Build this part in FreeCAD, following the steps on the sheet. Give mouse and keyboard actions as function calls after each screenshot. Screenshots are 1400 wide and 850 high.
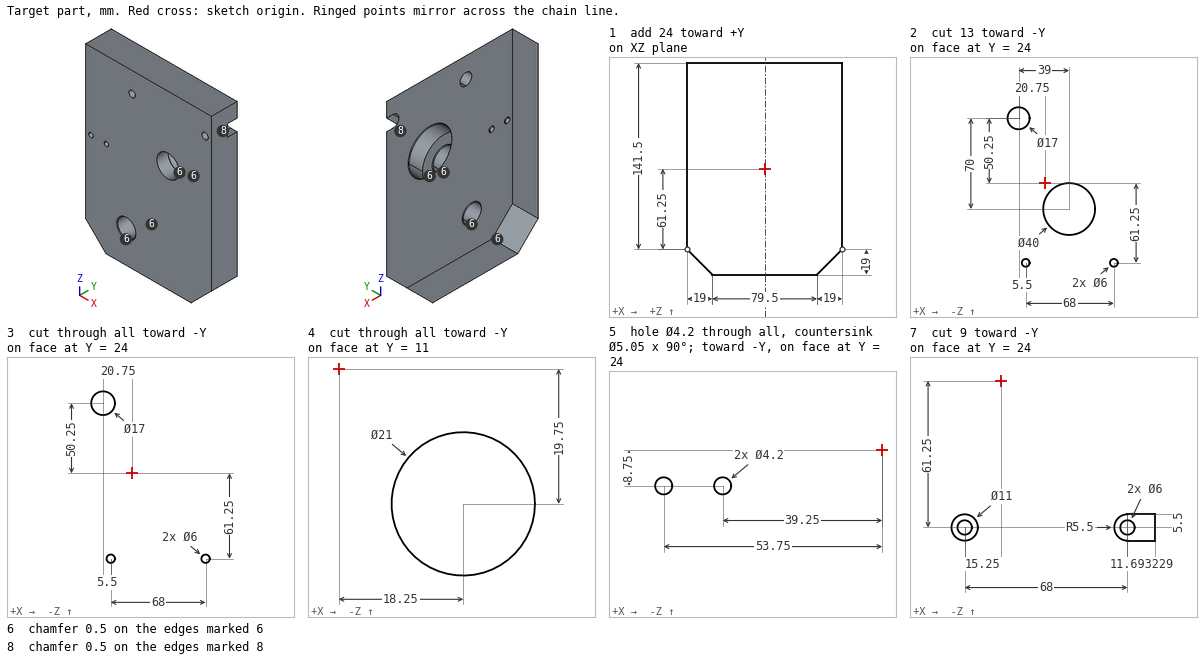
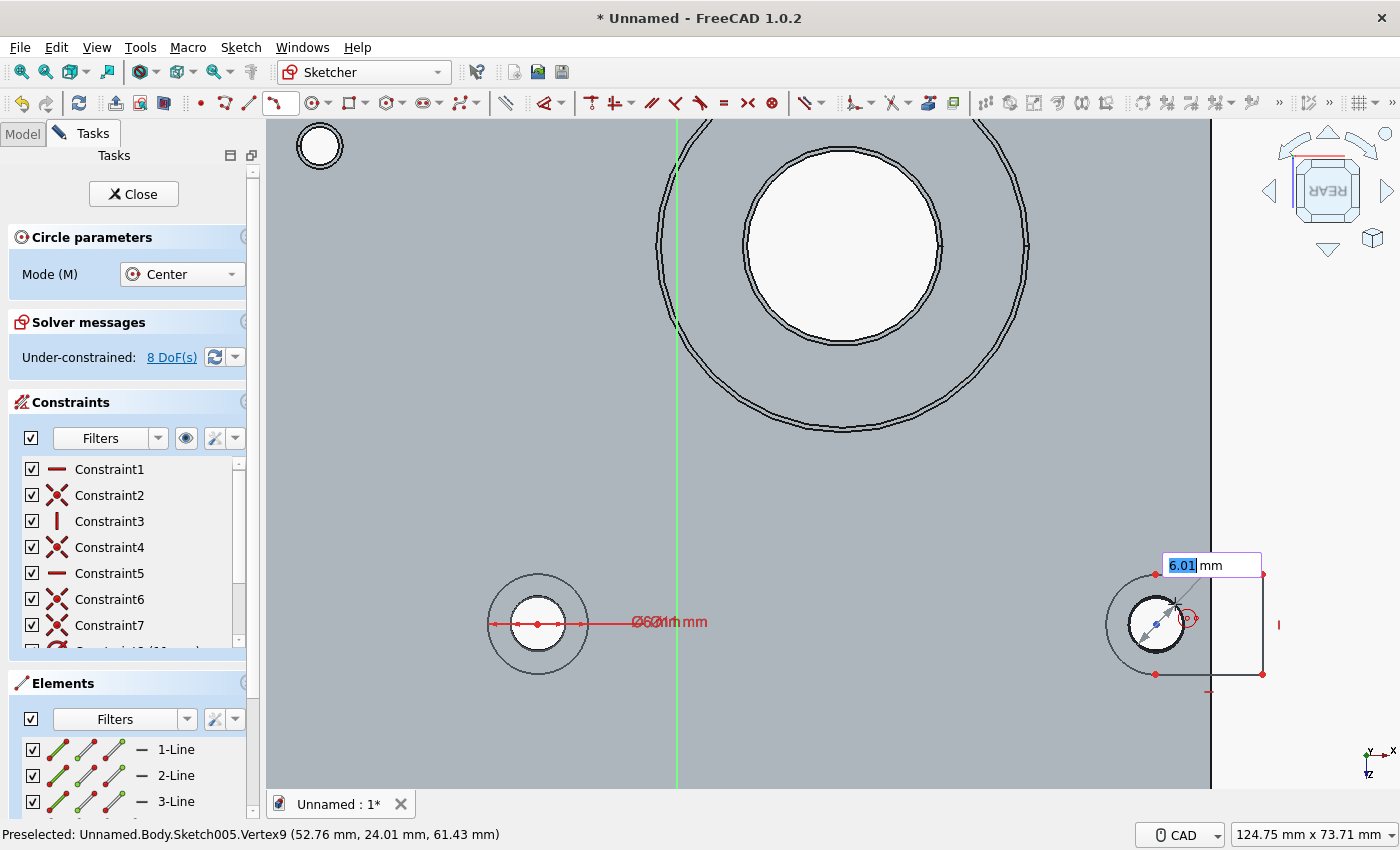
text(6)
key(Return)
key(Escape)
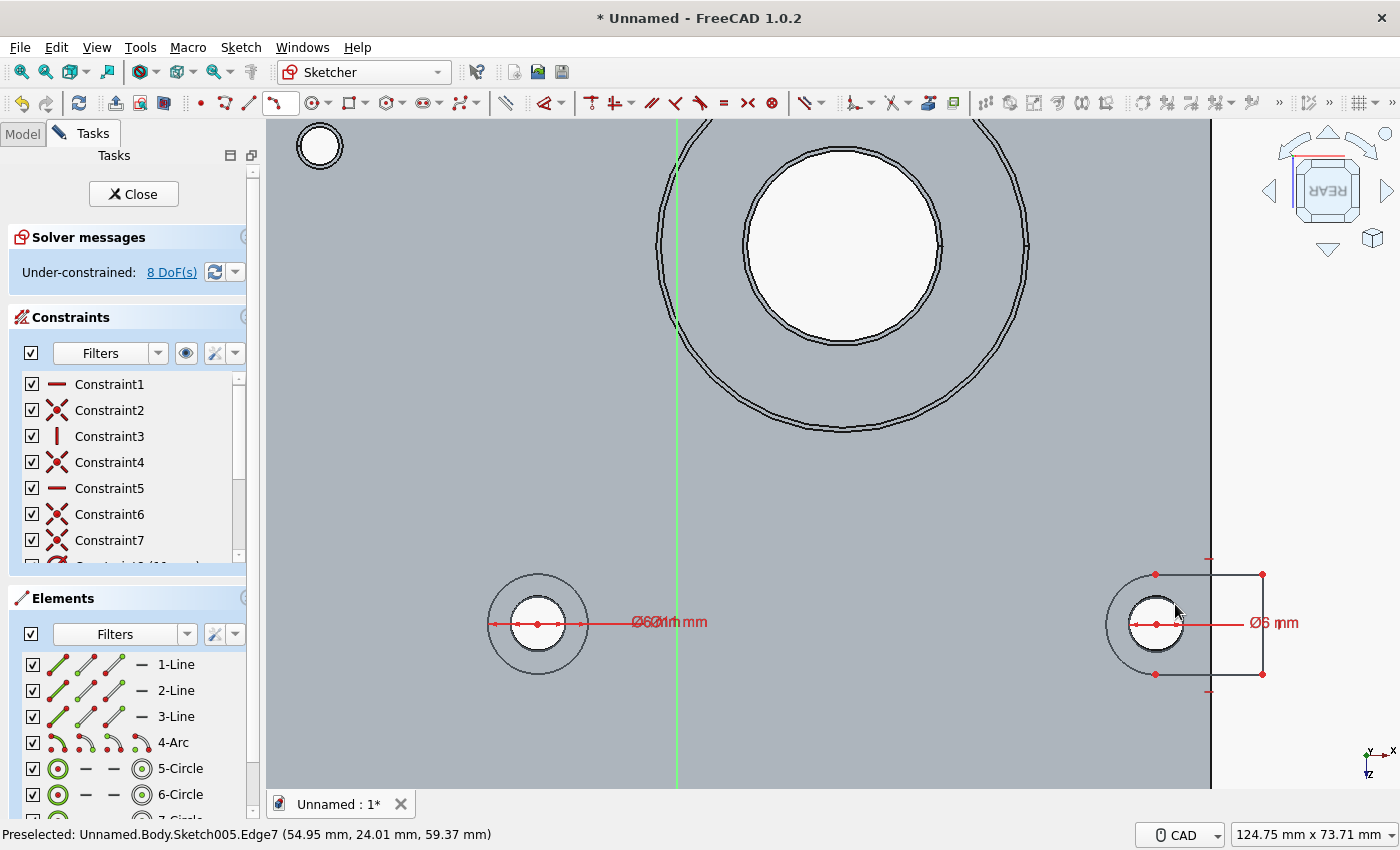
click(1188, 575)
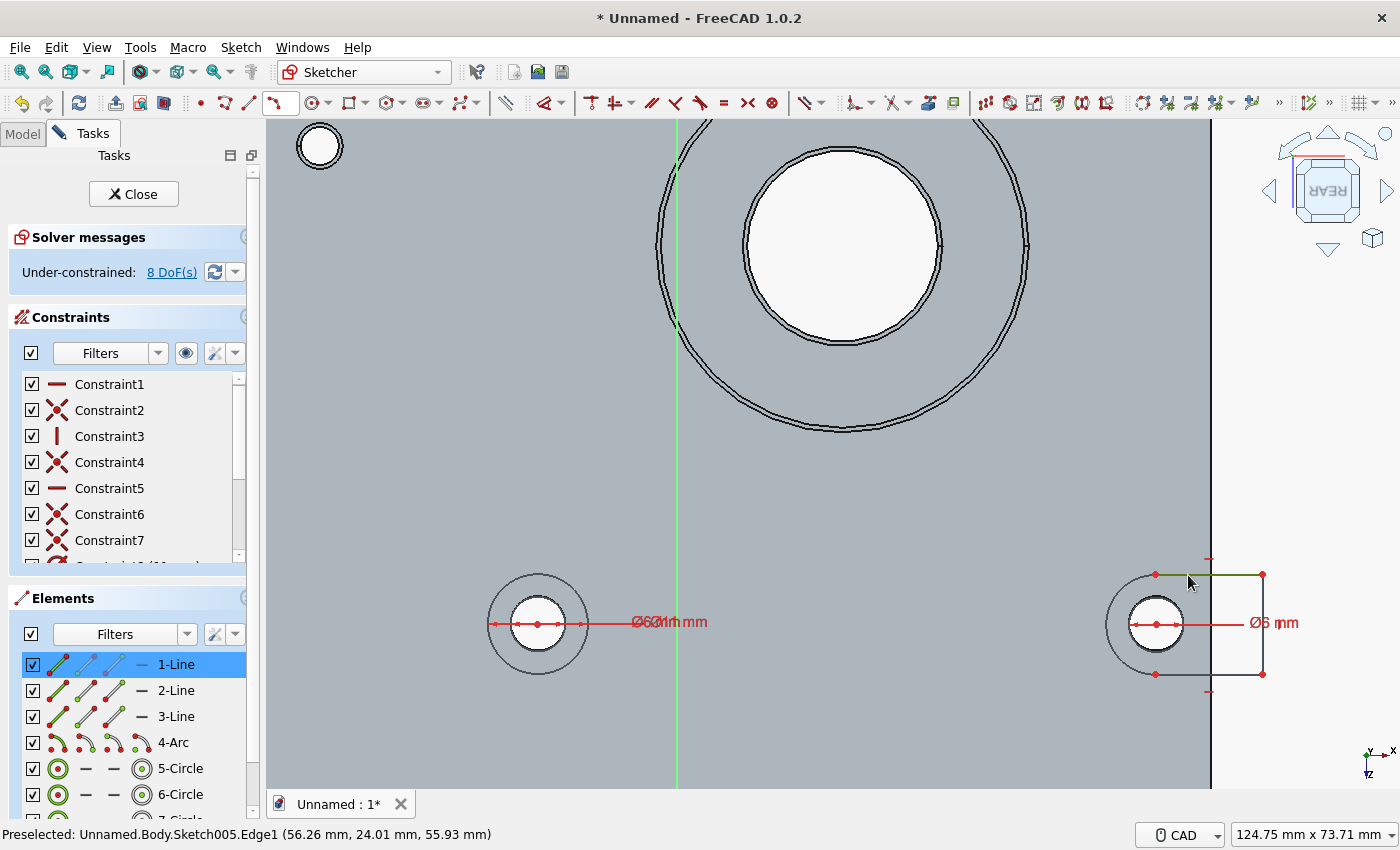
click(1116, 596)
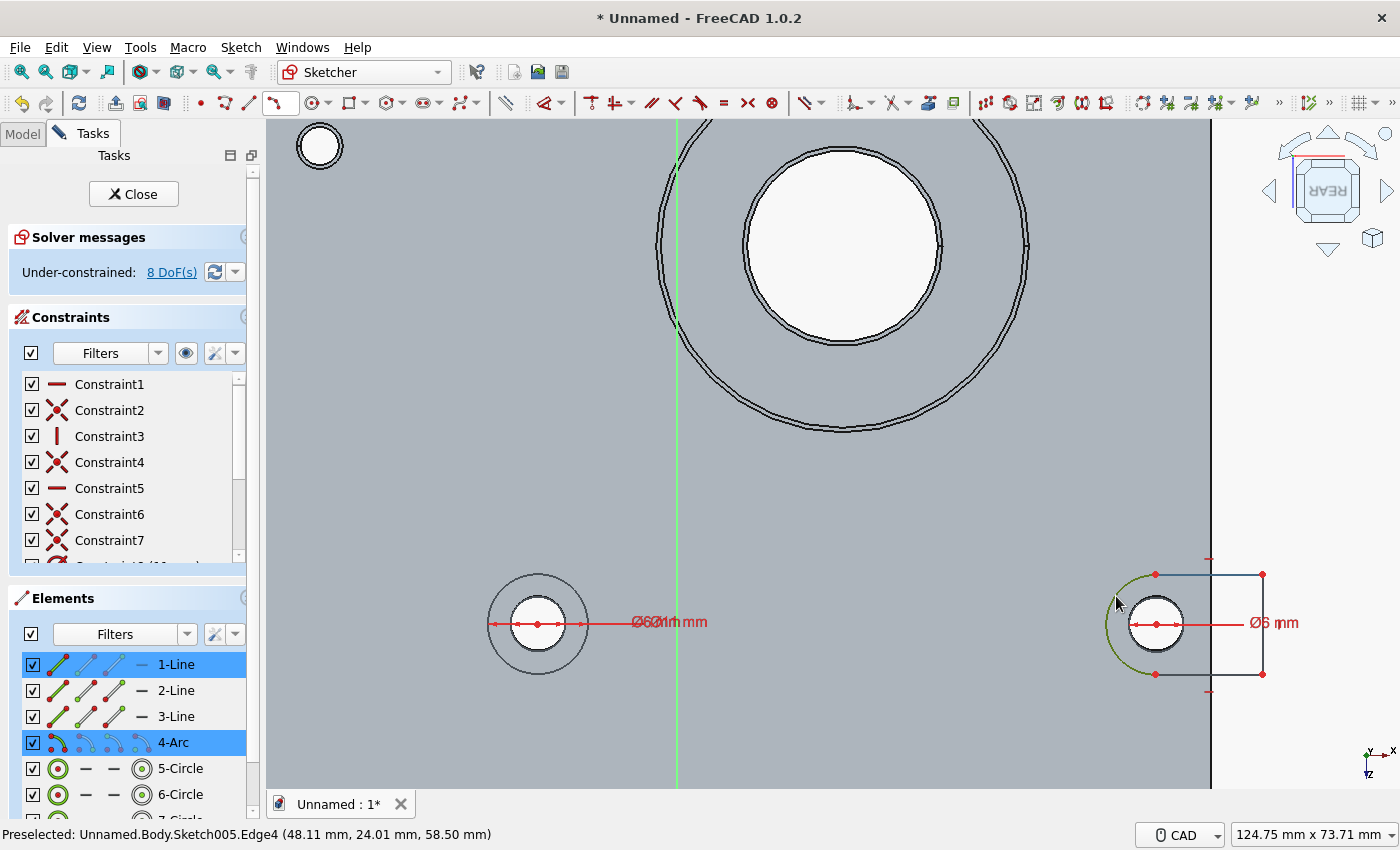
key(t)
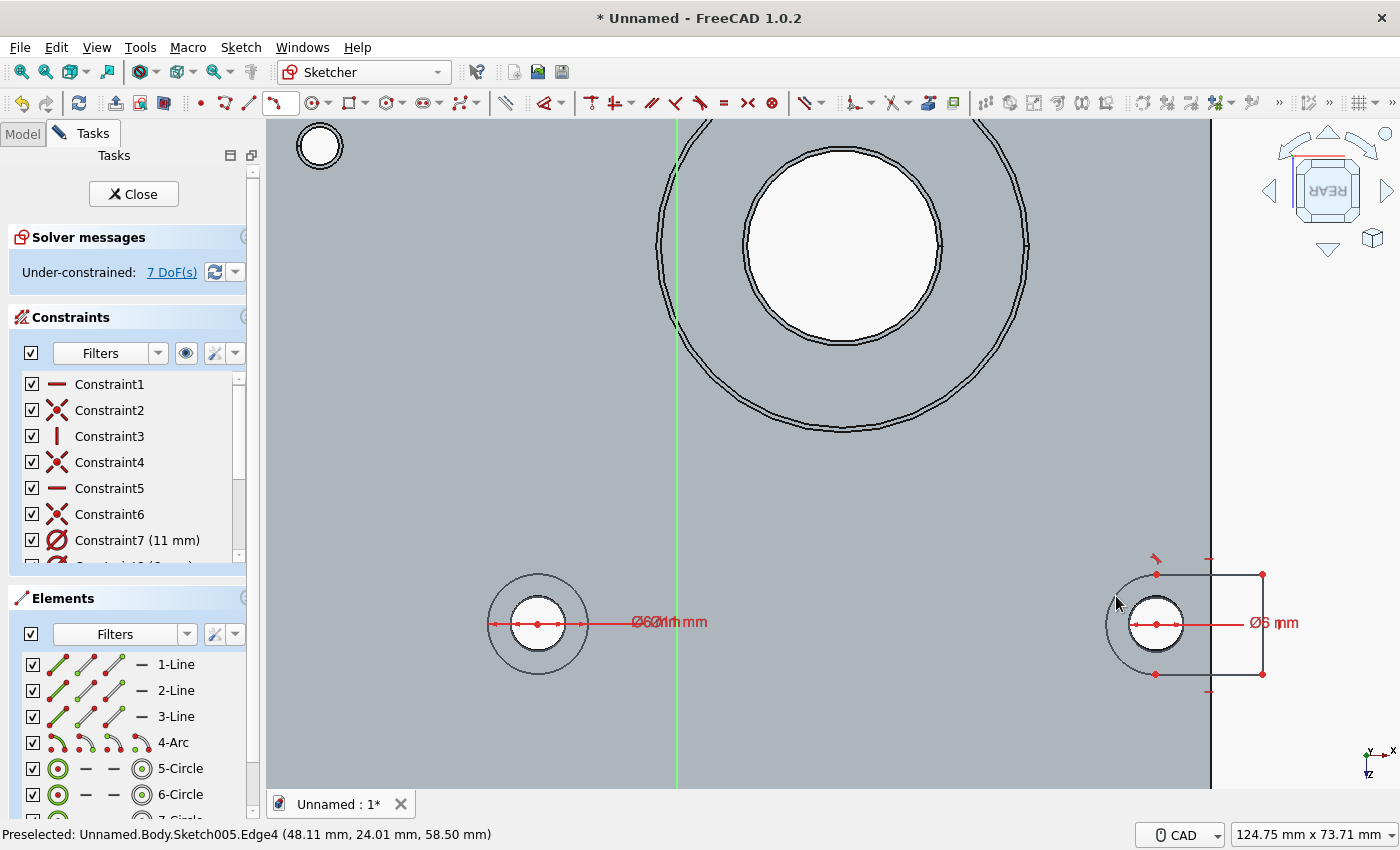
click(1231, 675)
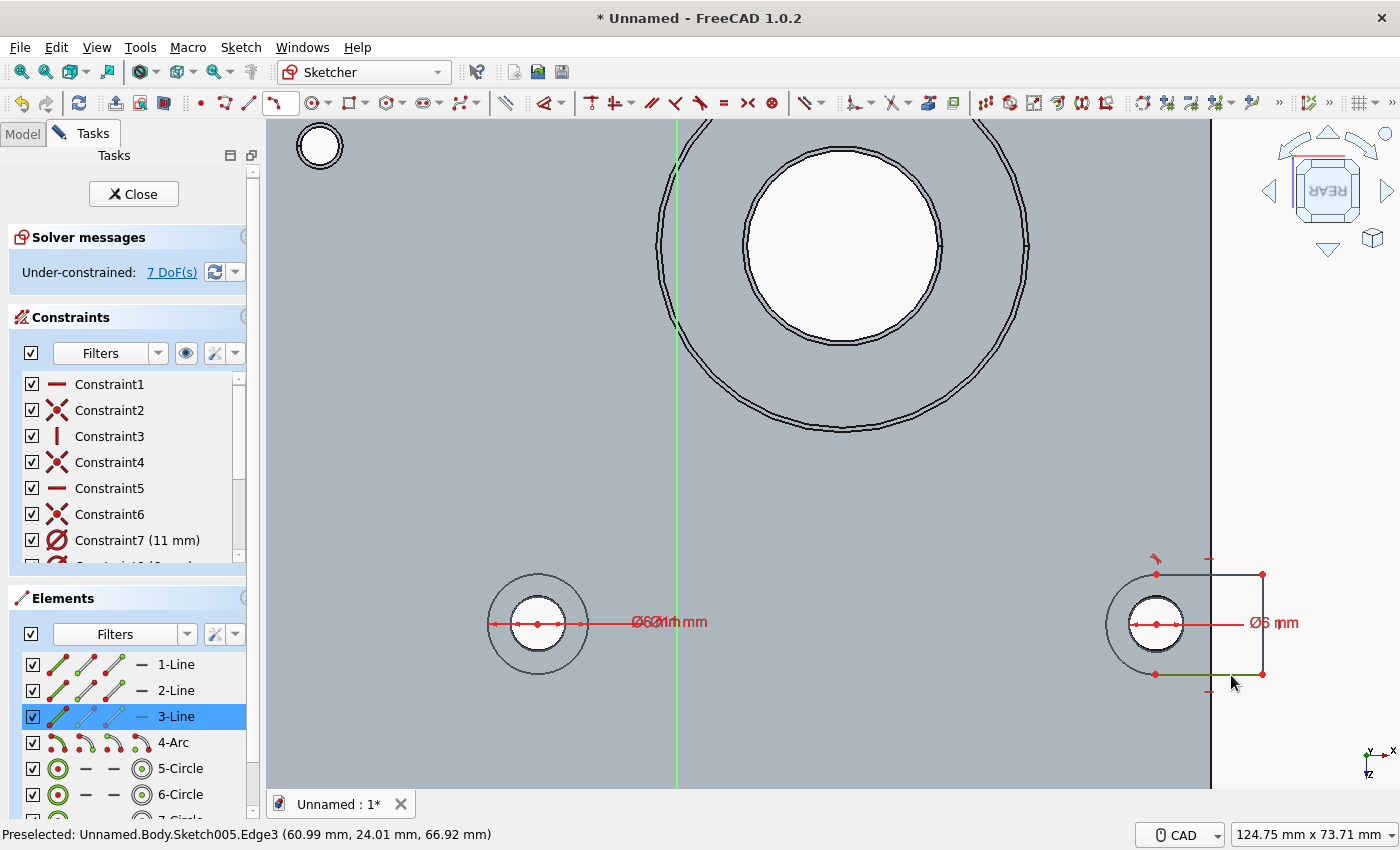
click(1116, 595)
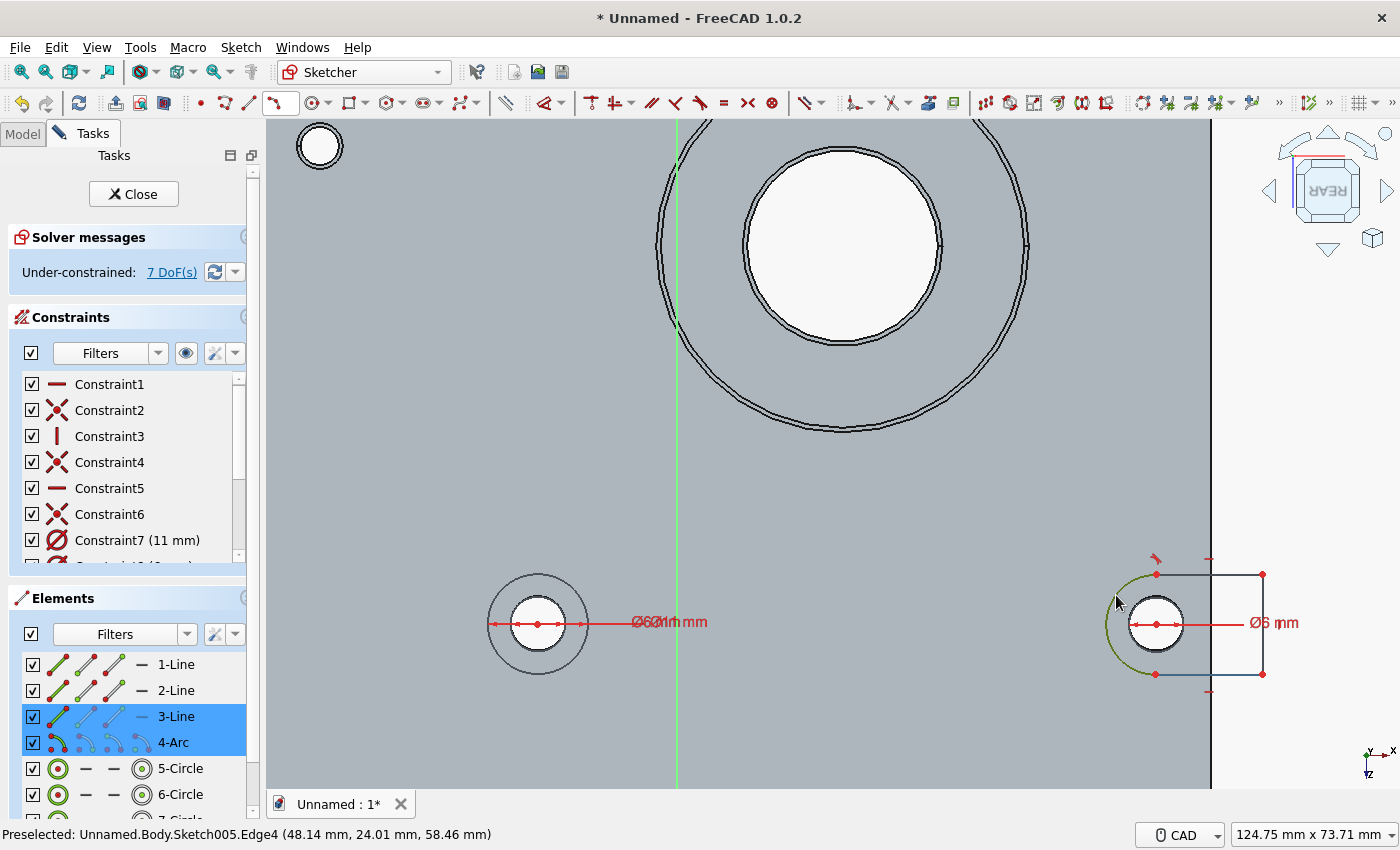
key(t)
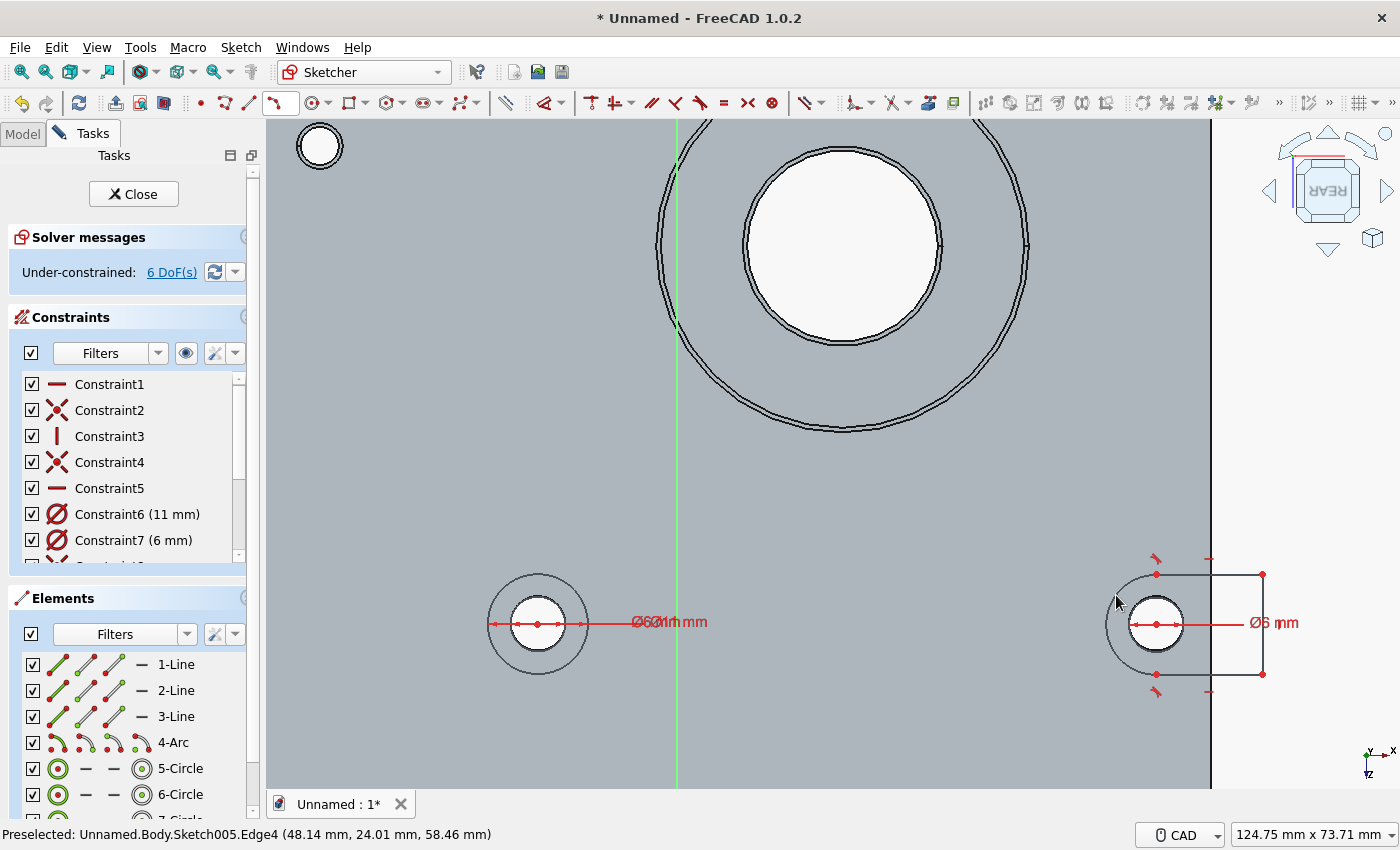
key(d)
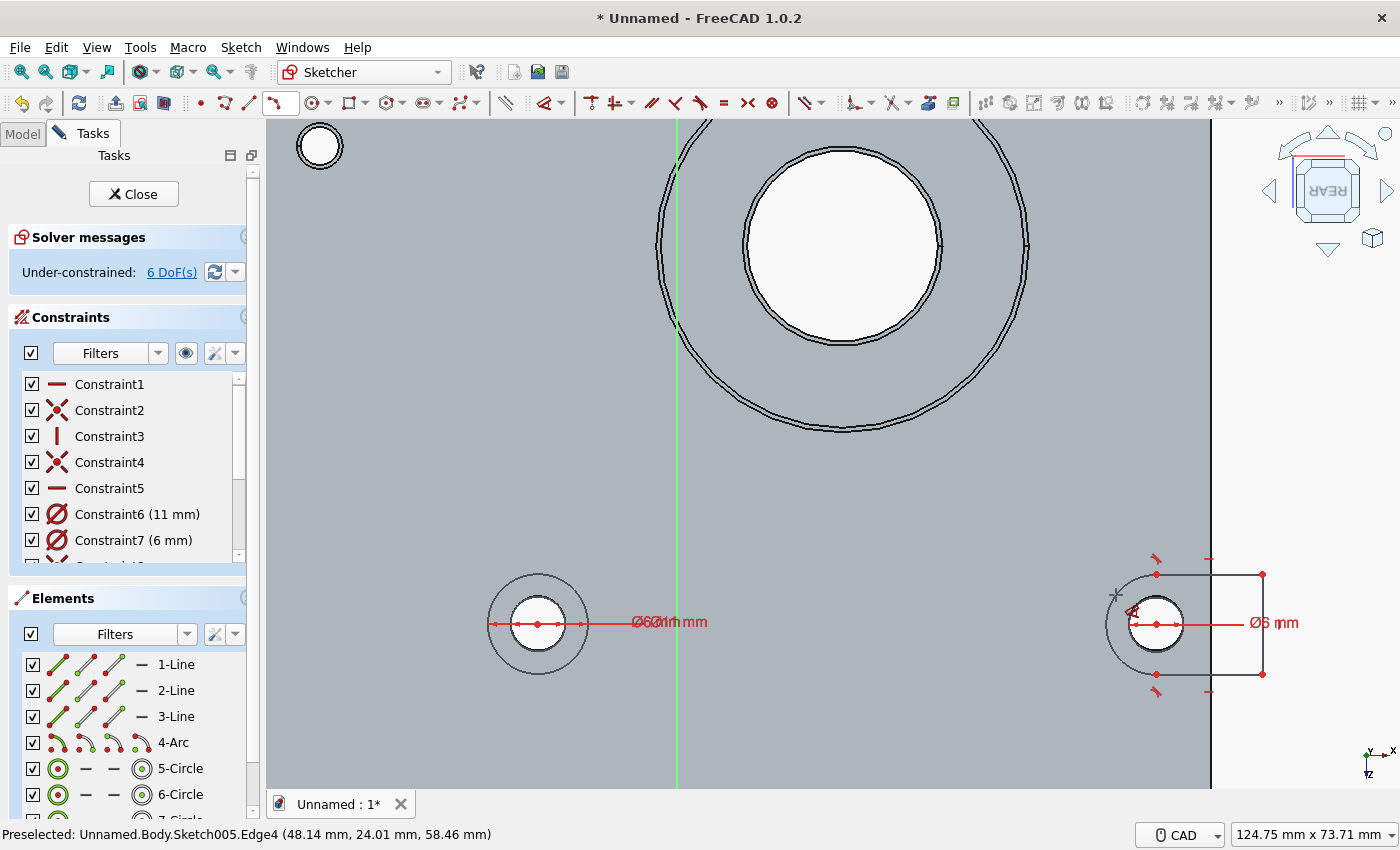
click(1116, 595)
click(1090, 576)